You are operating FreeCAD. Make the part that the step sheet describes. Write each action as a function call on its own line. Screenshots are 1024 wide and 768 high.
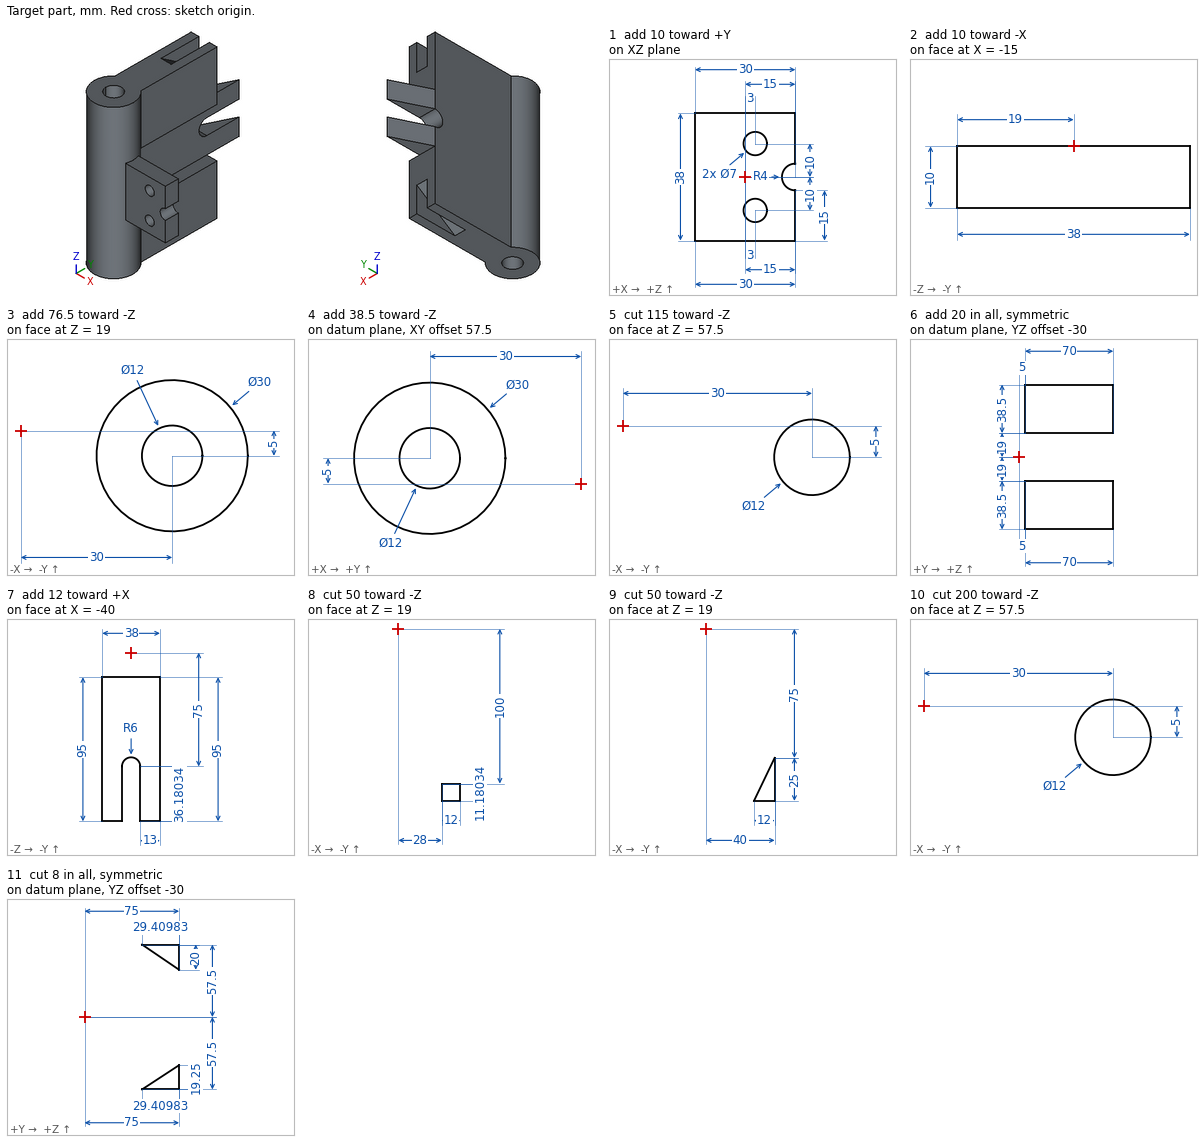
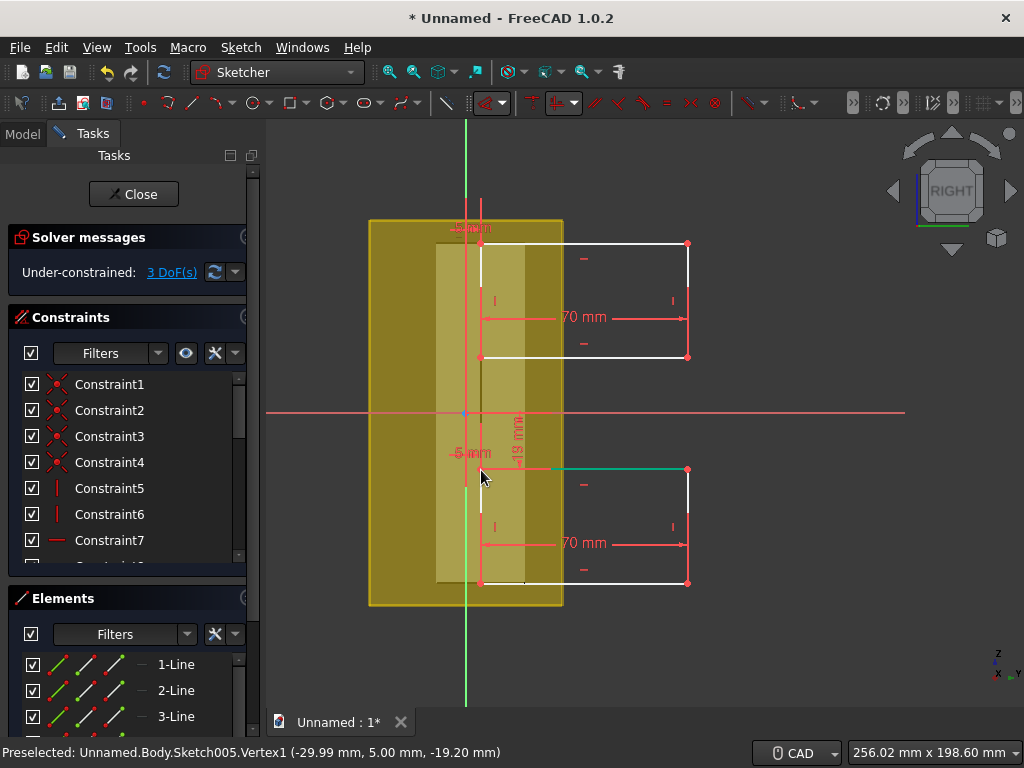
click(481, 358)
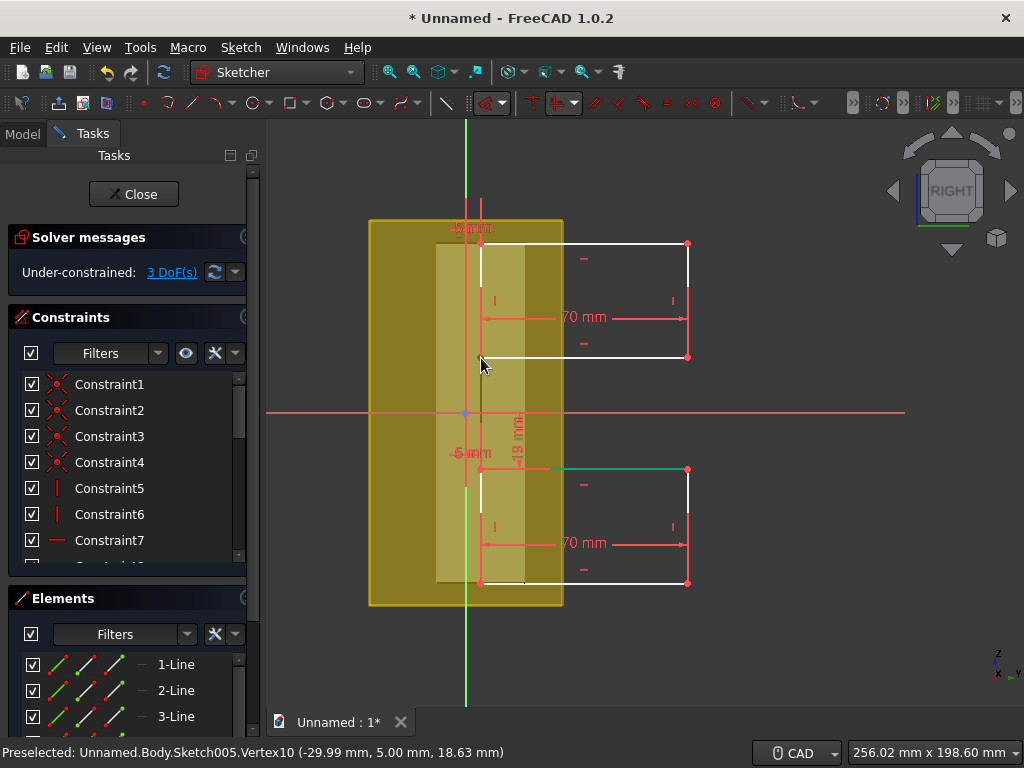
click(504, 104)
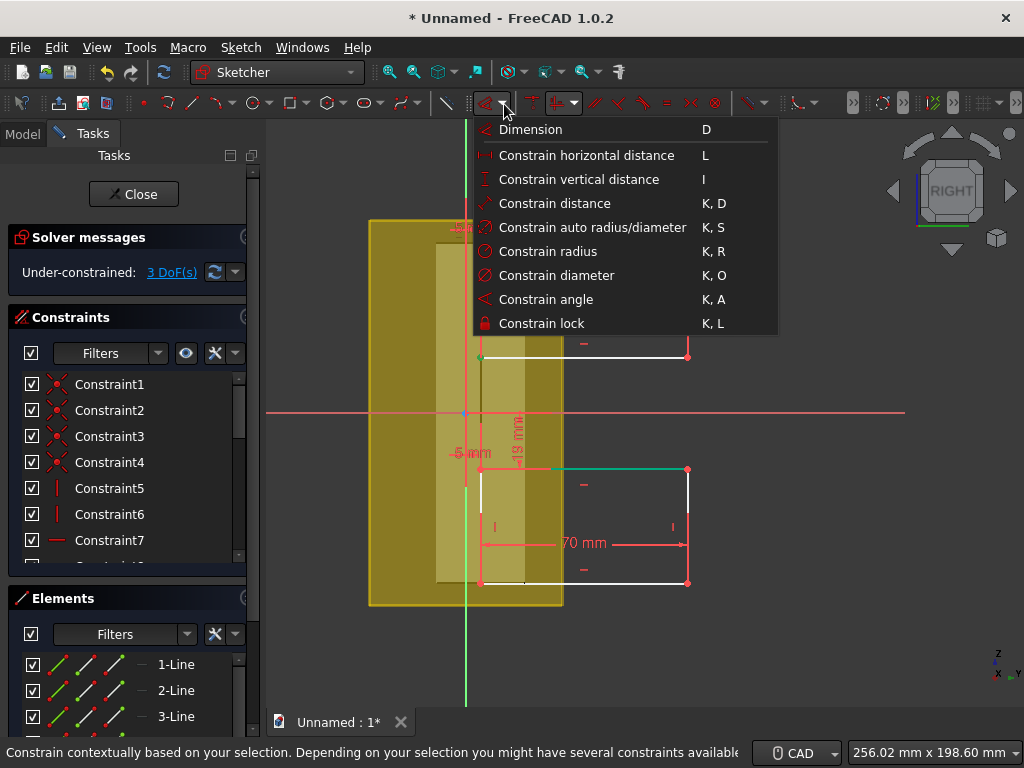
click(626, 179)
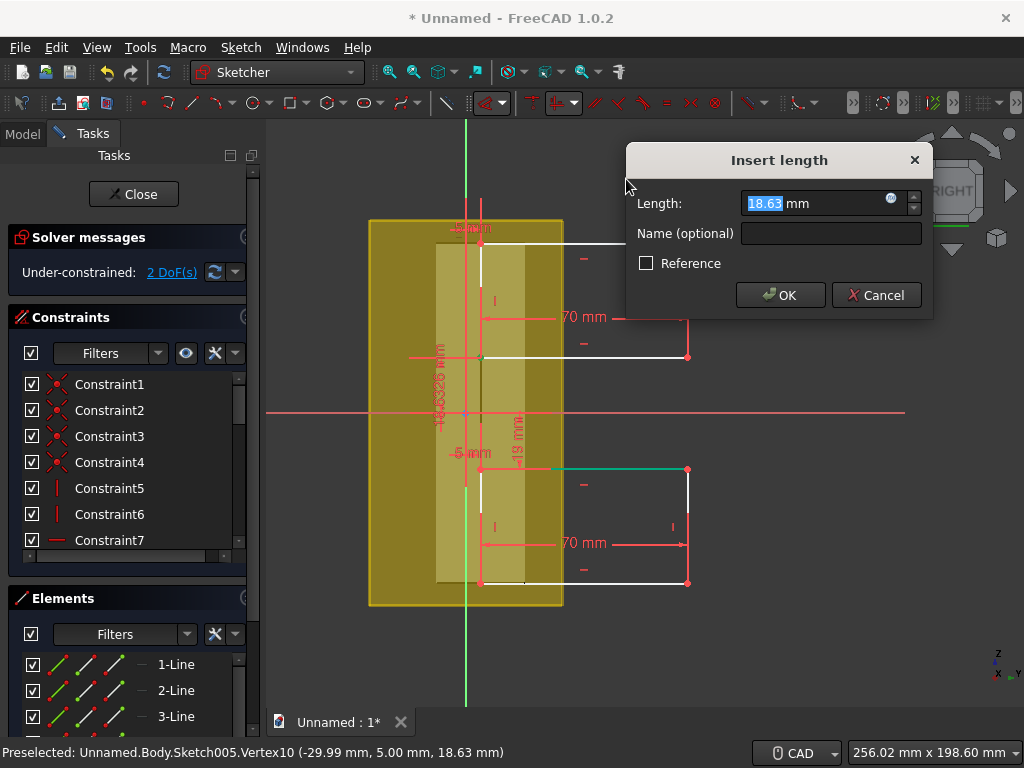
text(19)
key(Return)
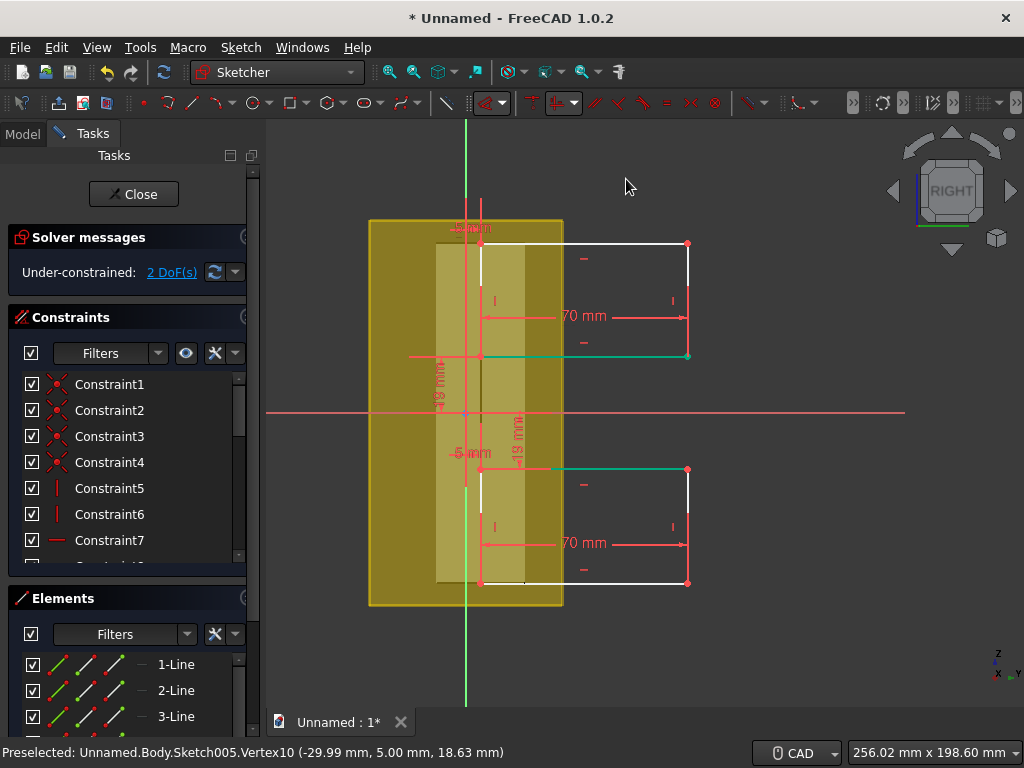
click(481, 504)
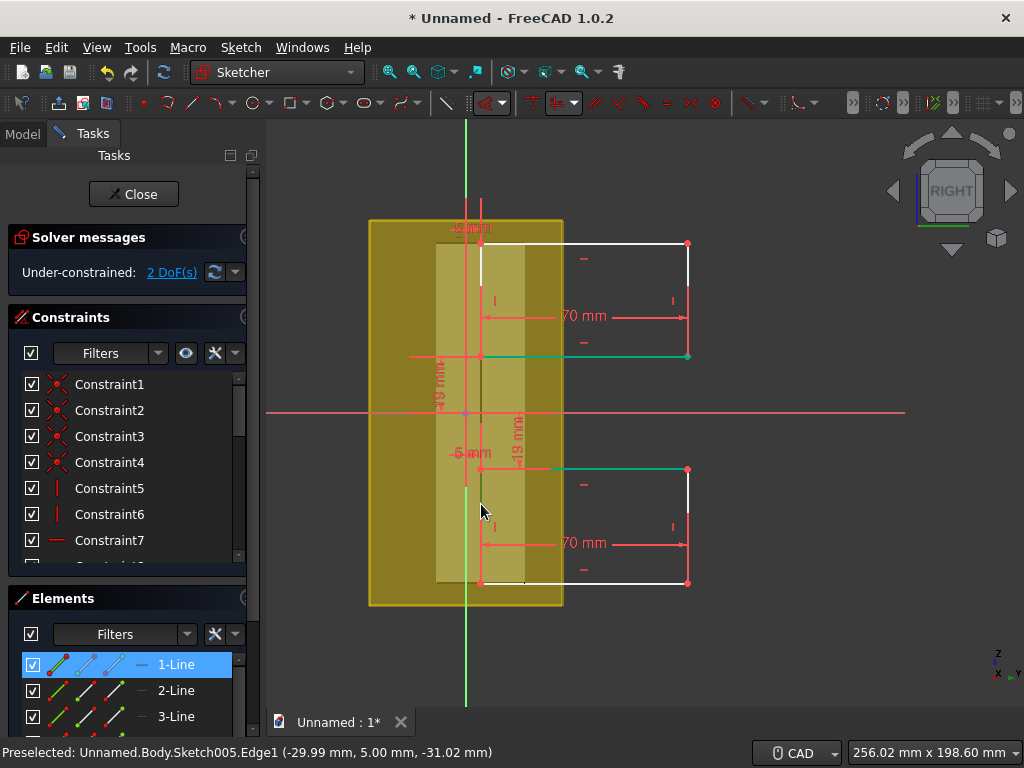
key(i)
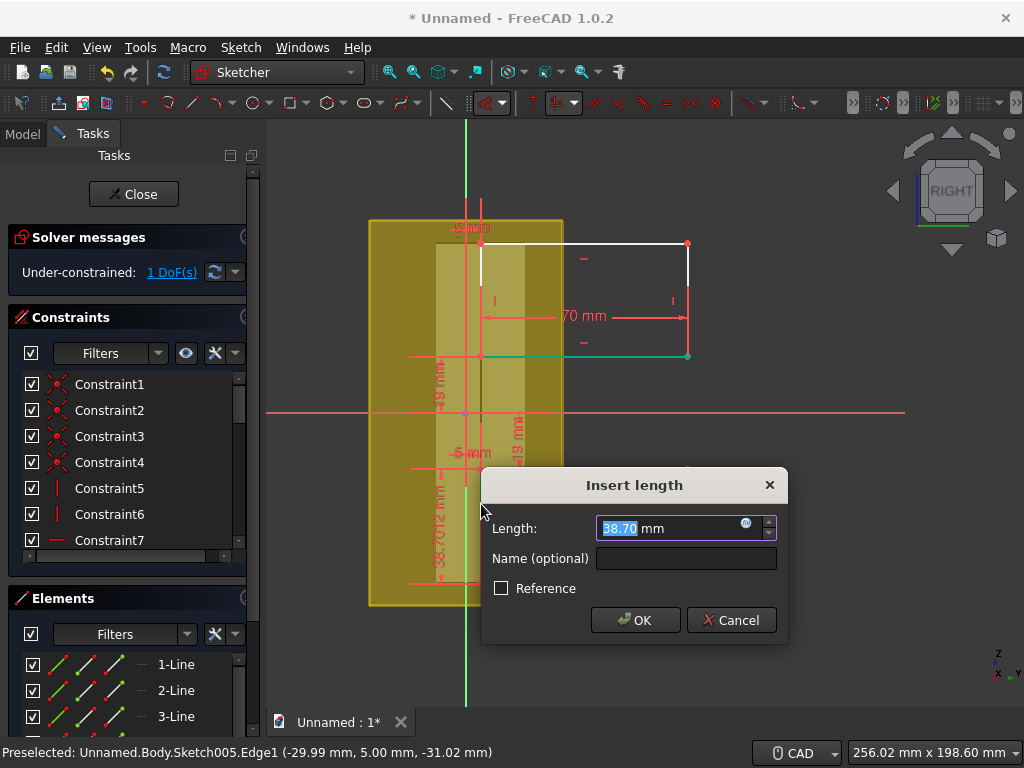
text(38.5)
key(Return)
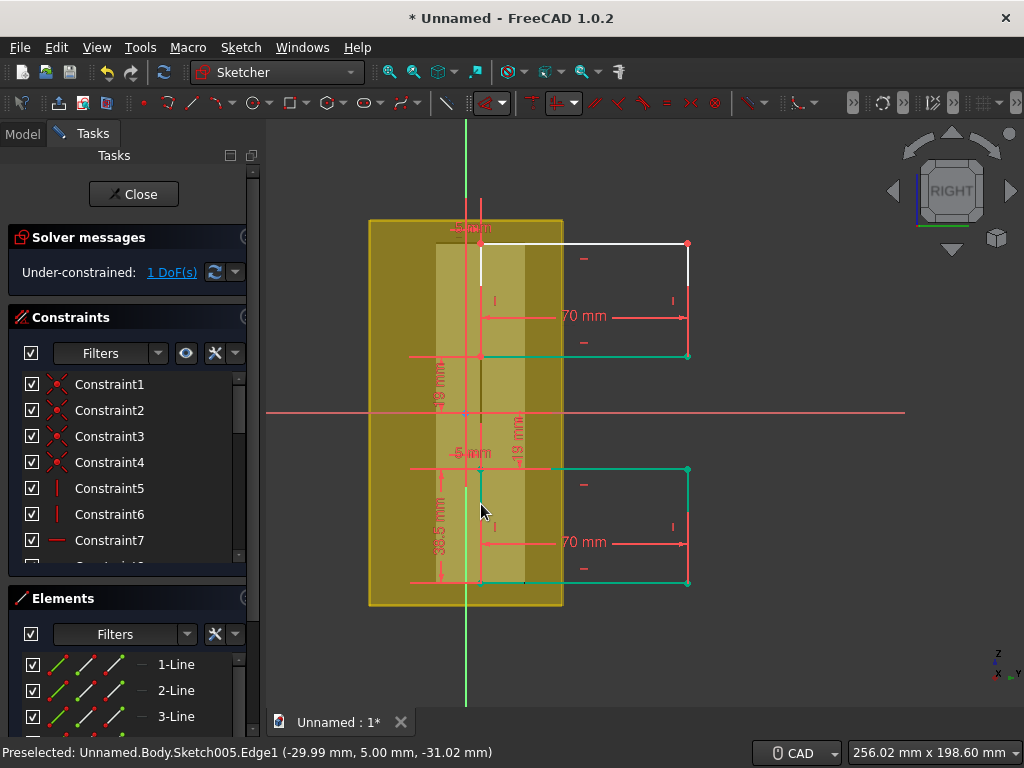
click(481, 278)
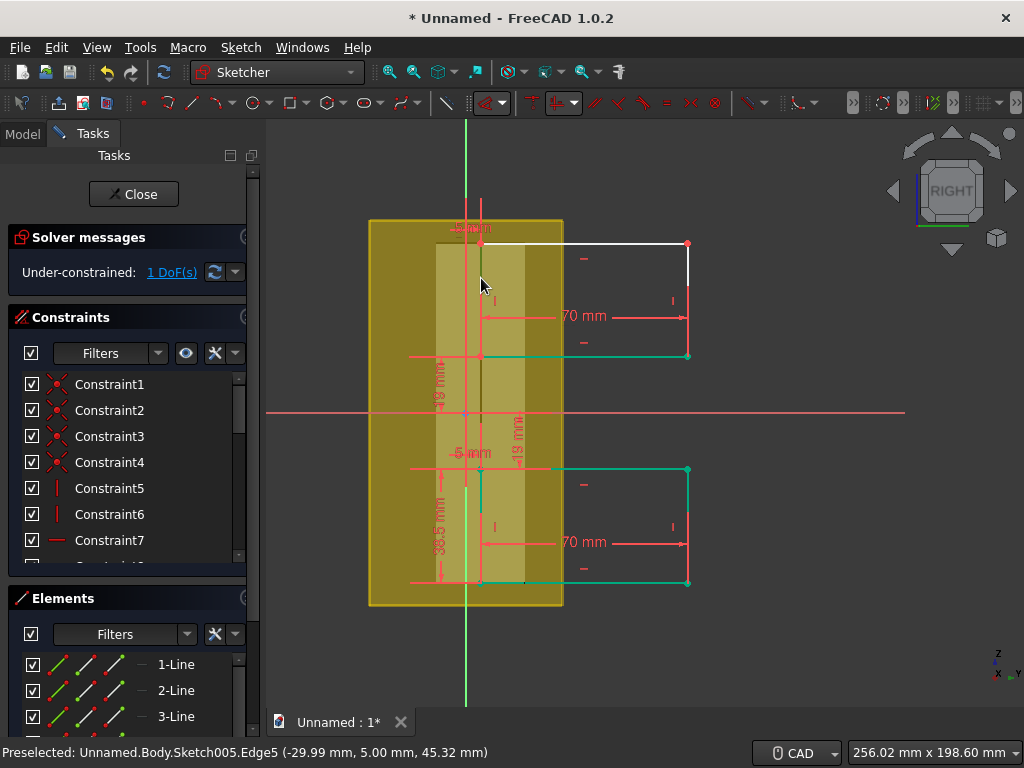
click(504, 104)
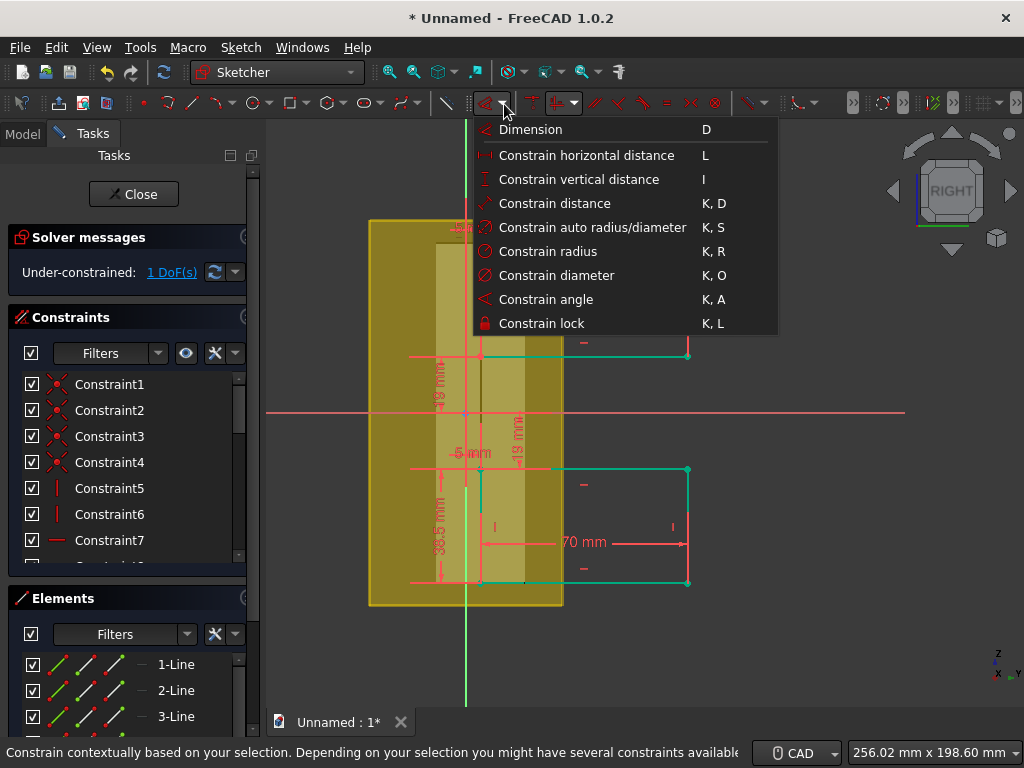
click(626, 179)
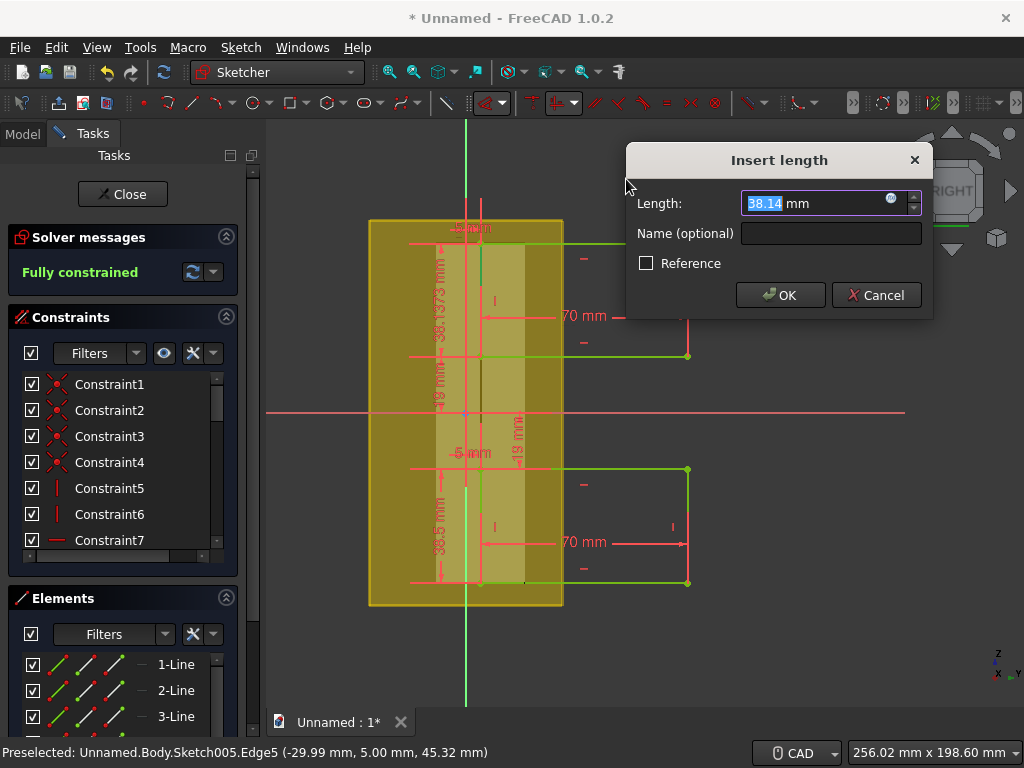
text(38.5)
key(Return)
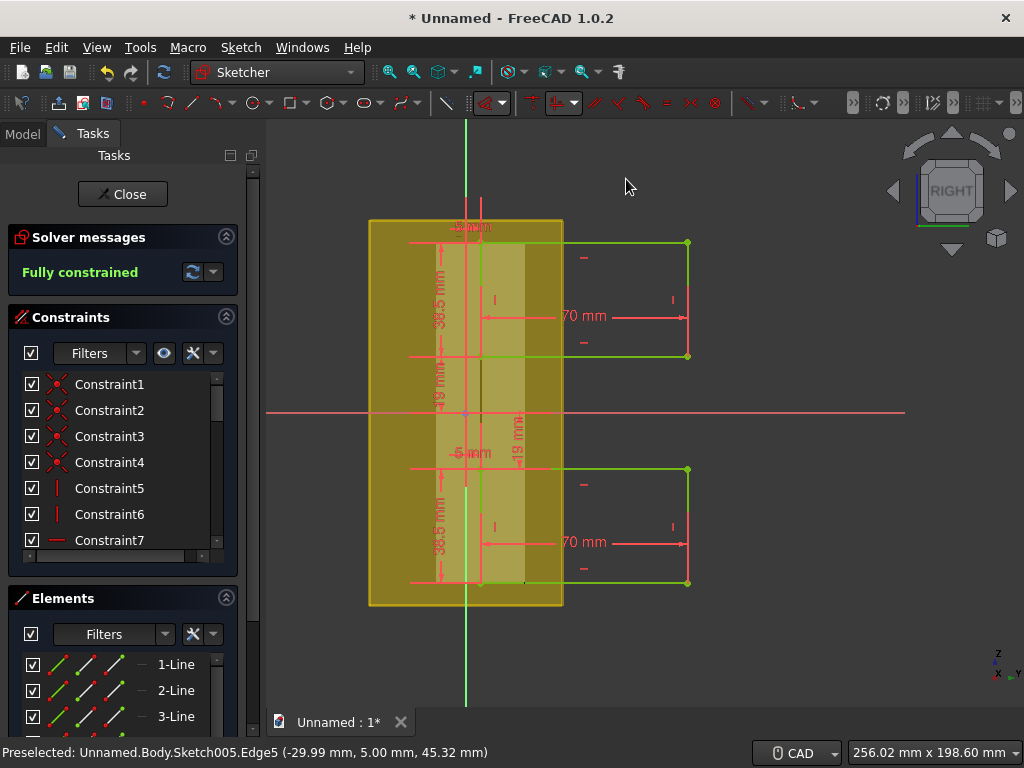
click(123, 194)